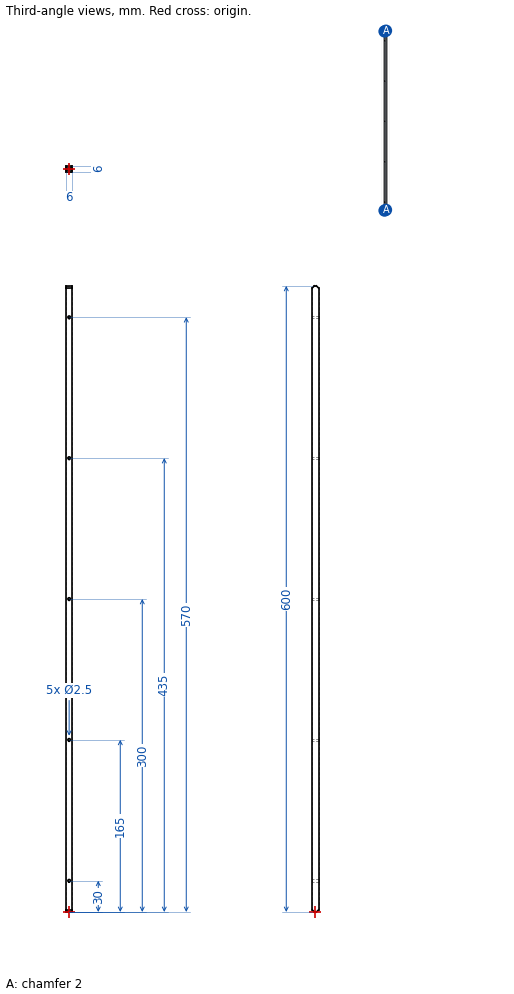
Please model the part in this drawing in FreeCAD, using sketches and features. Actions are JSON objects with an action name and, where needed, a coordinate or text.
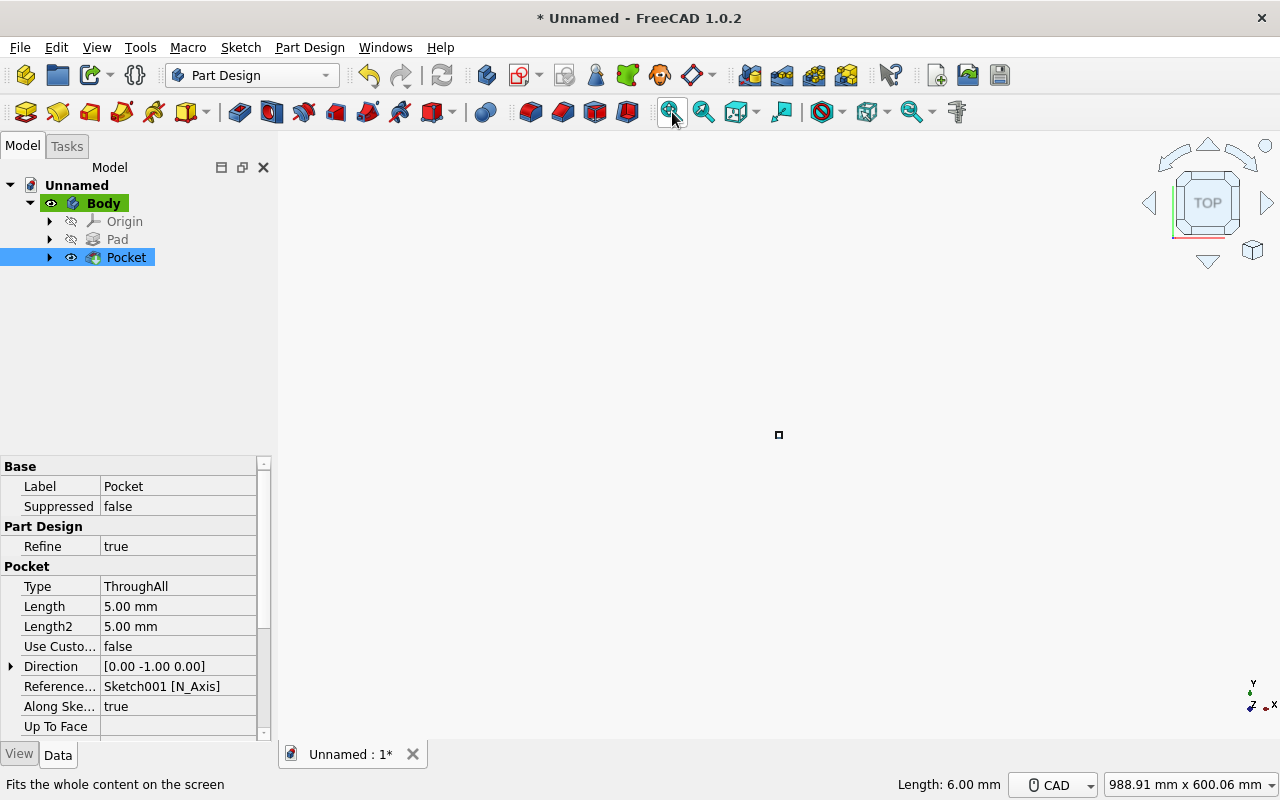
{"action": "left_click", "coordinate": [672, 112]}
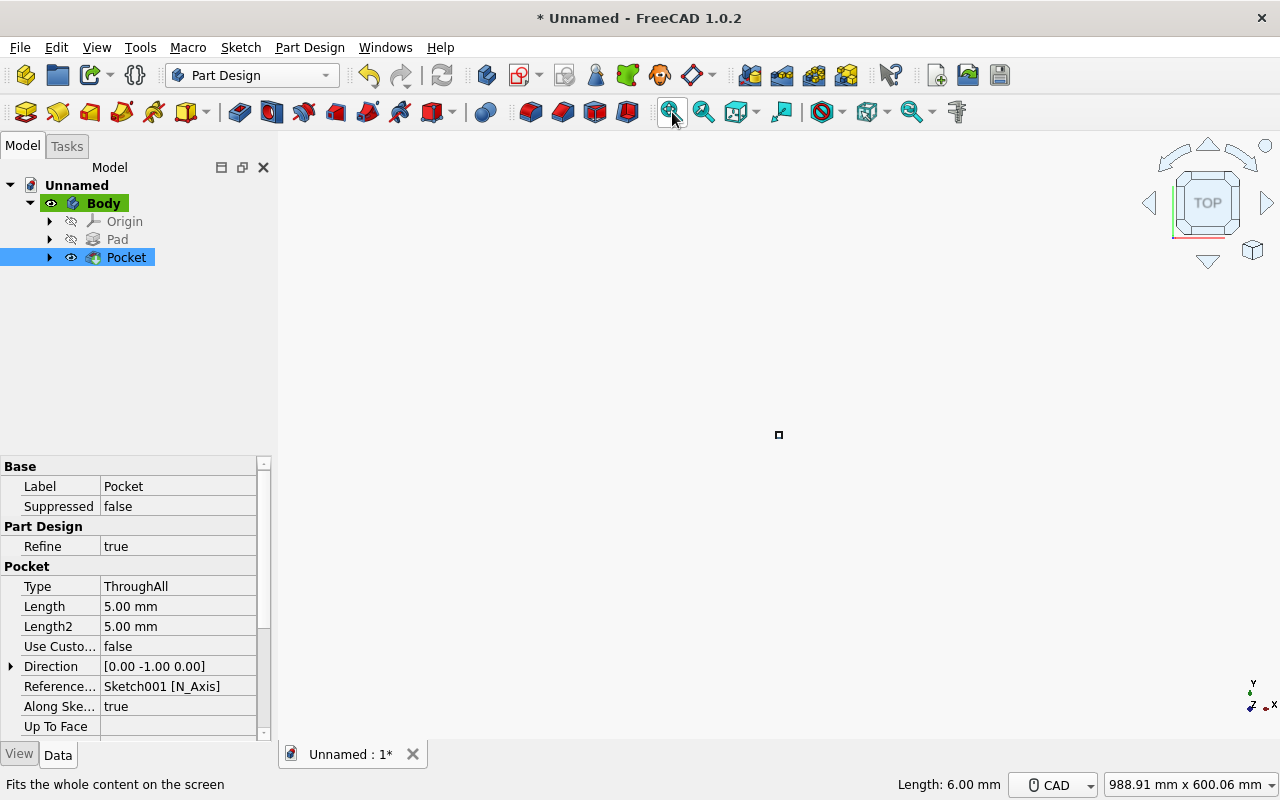
{"action": "scroll", "coordinate": [779, 437], "scroll_direction": "up", "scroll_amount": 10}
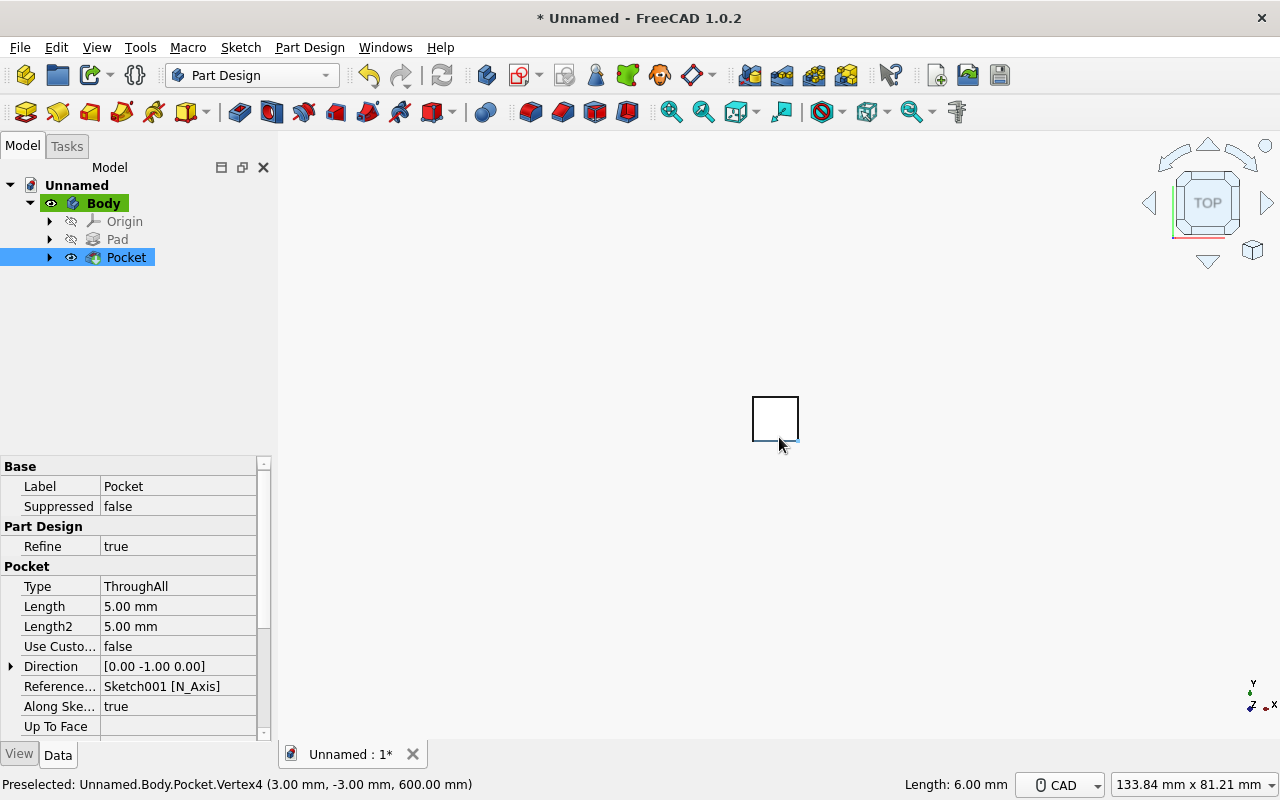
{"action": "left_click", "coordinate": [776, 396], "text": "ctrl"}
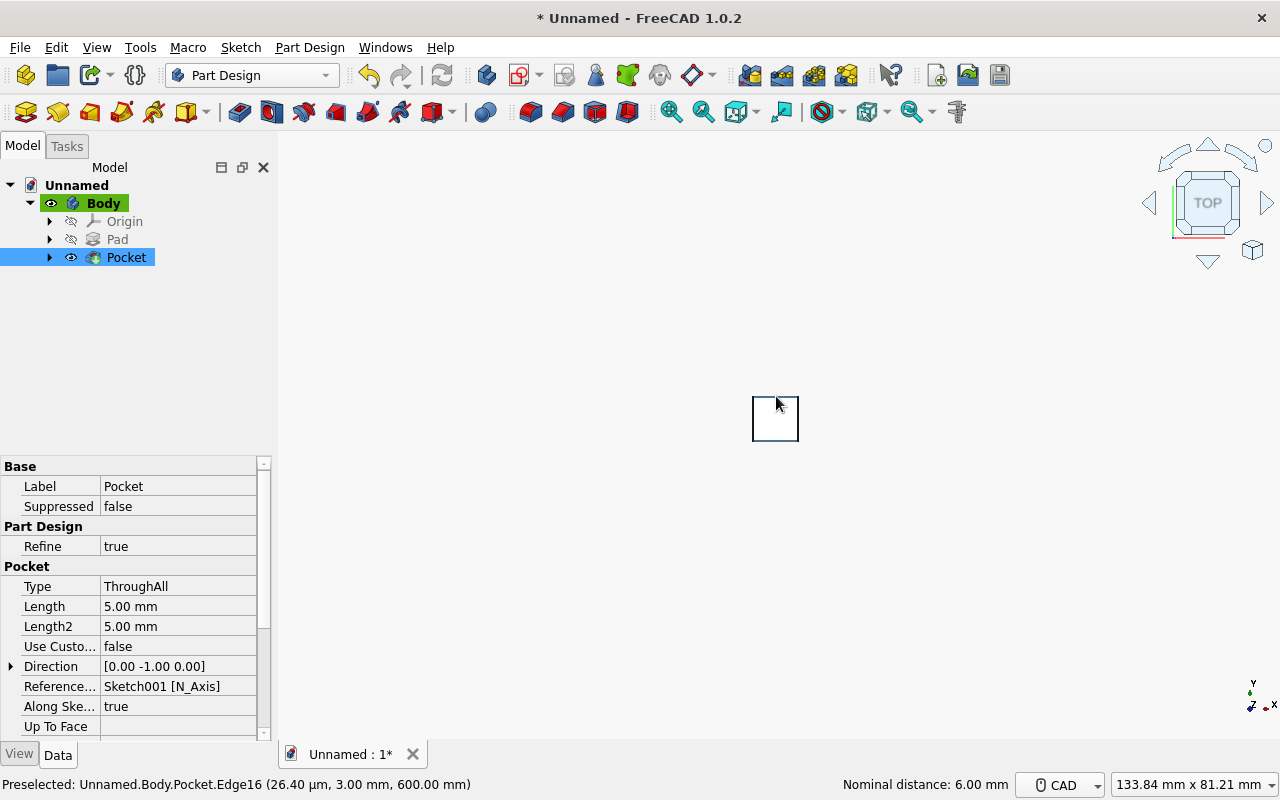
{"action": "left_click", "coordinate": [672, 112]}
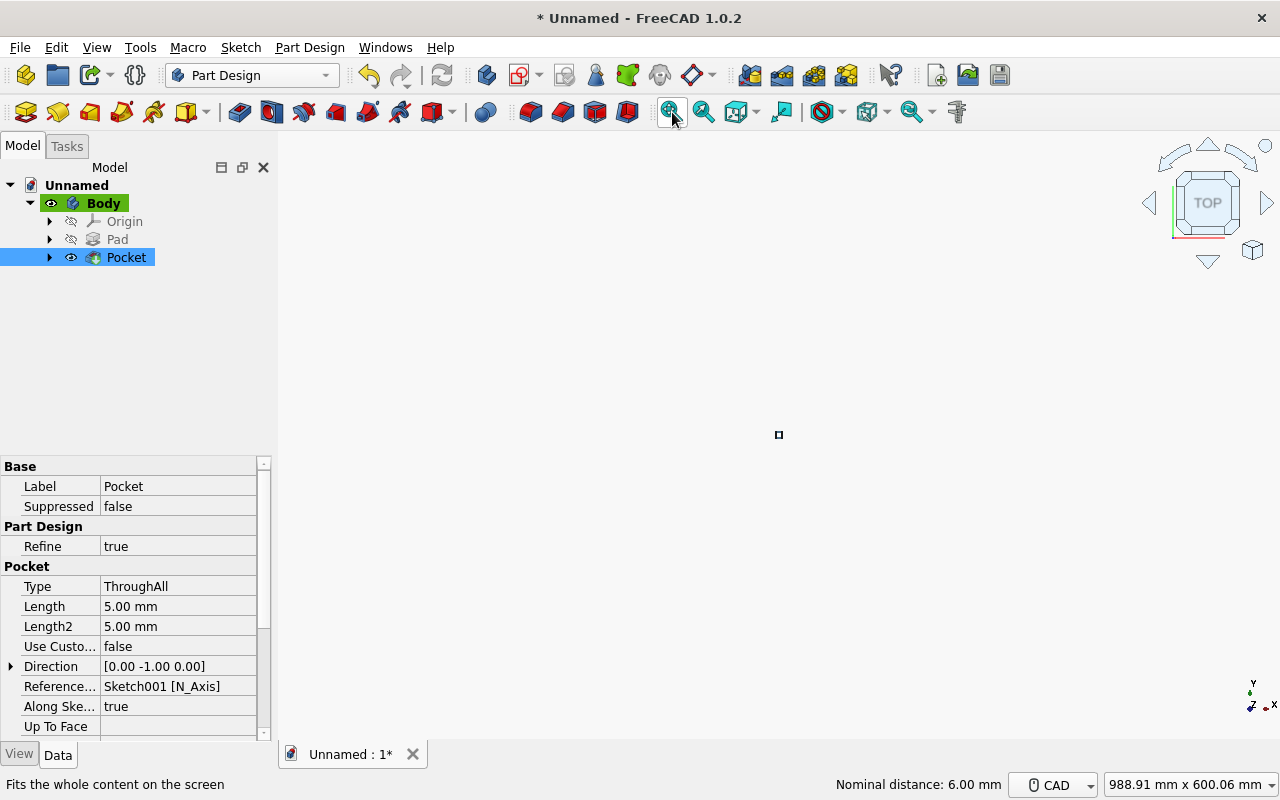
{"action": "key", "text": "1"}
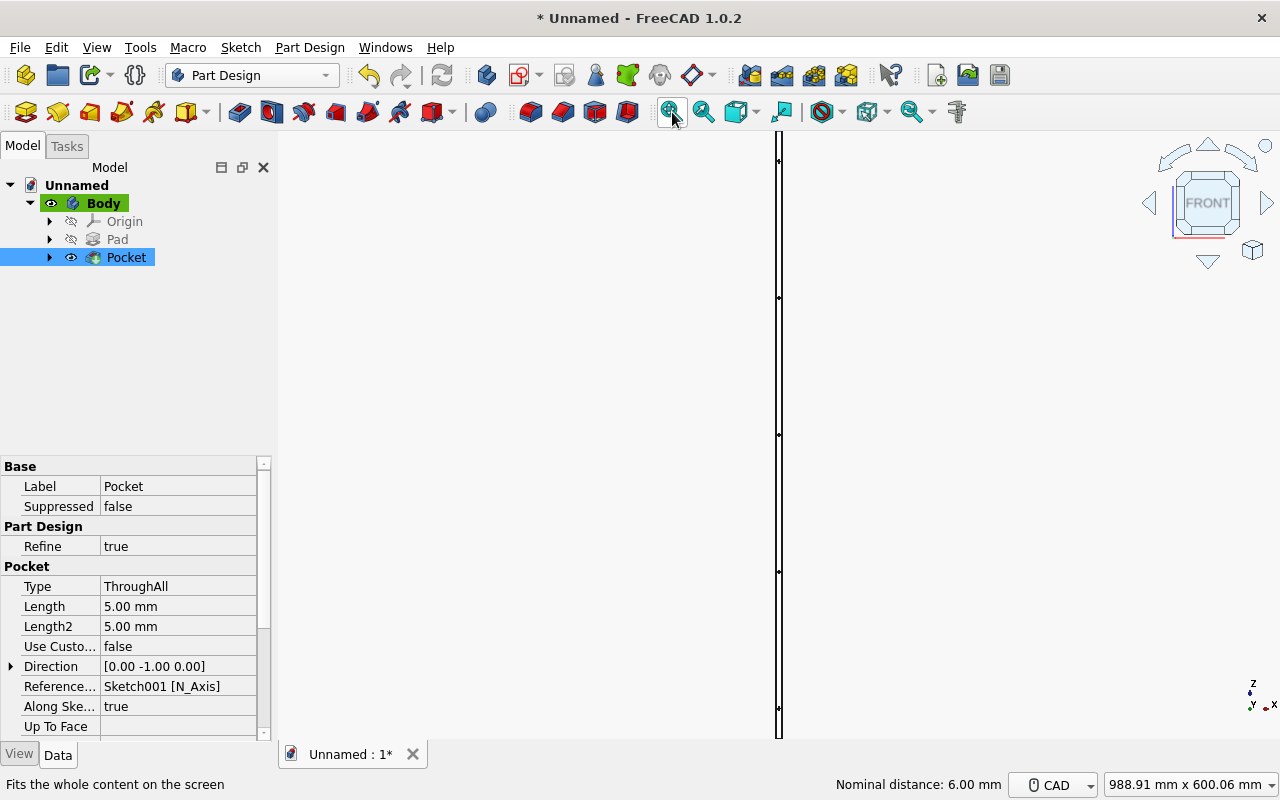
{"action": "left_click", "coordinate": [672, 112]}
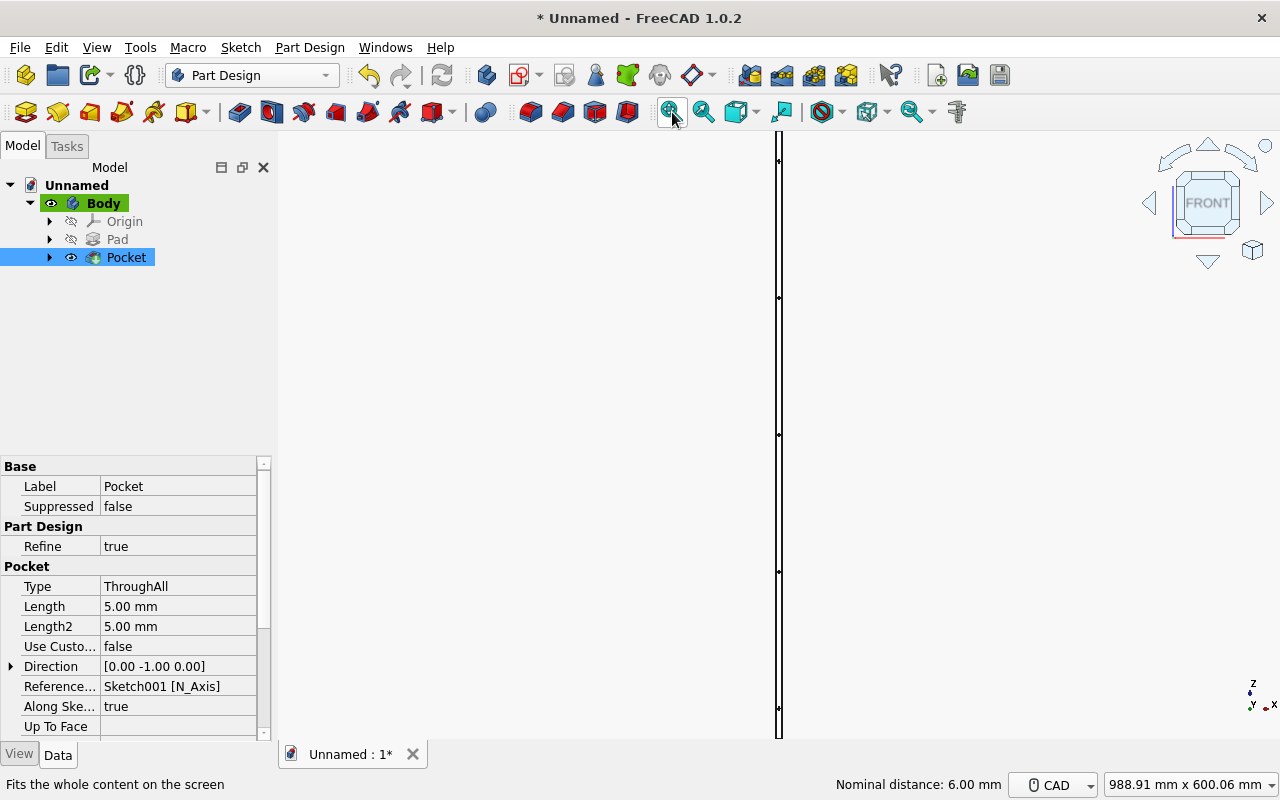
{"action": "key", "text": "3"}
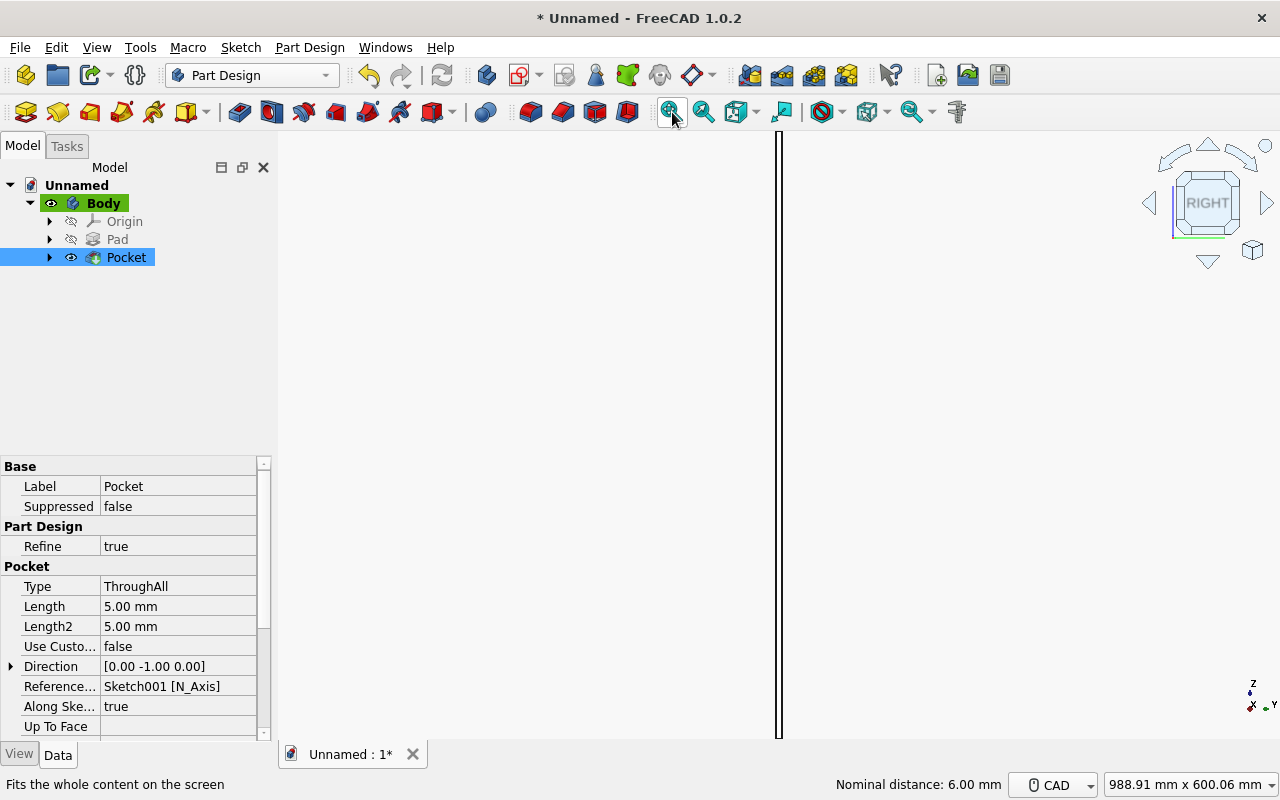
{"action": "left_click", "coordinate": [672, 112]}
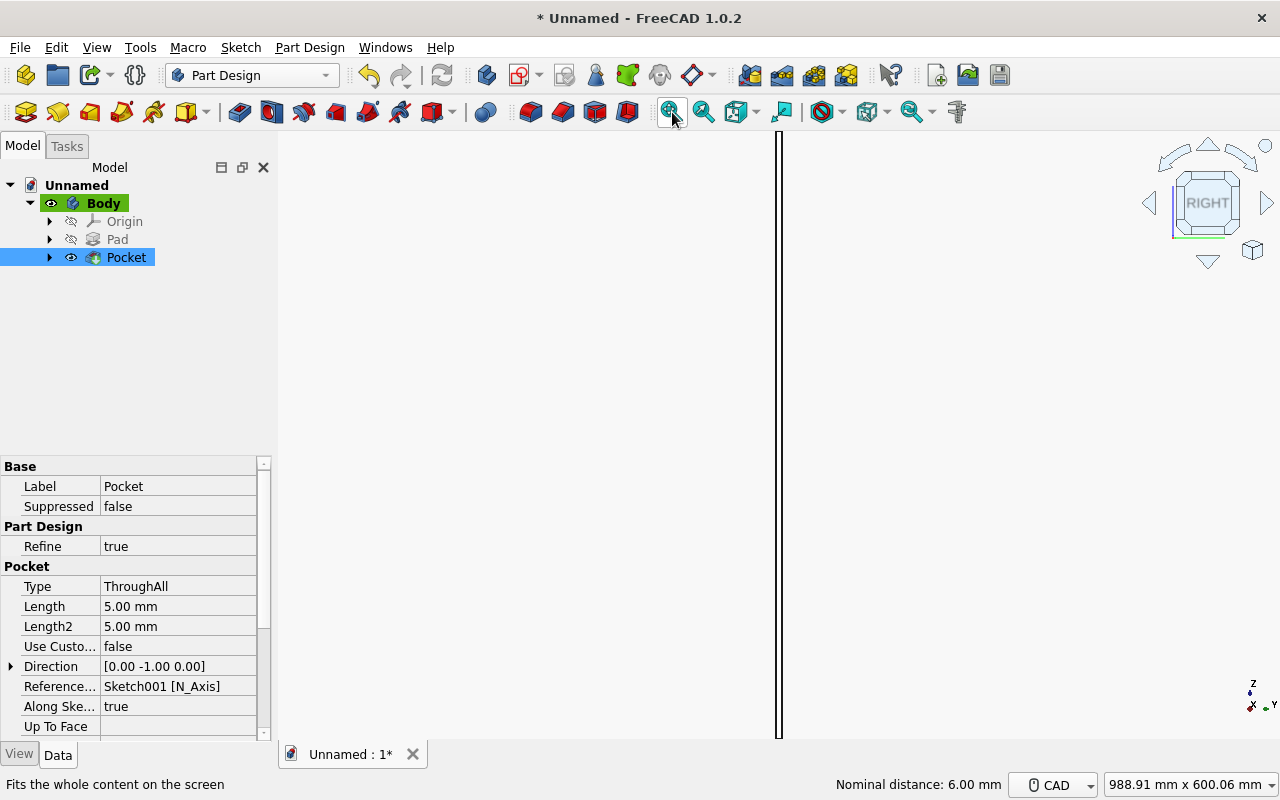
{"action": "key", "text": "5"}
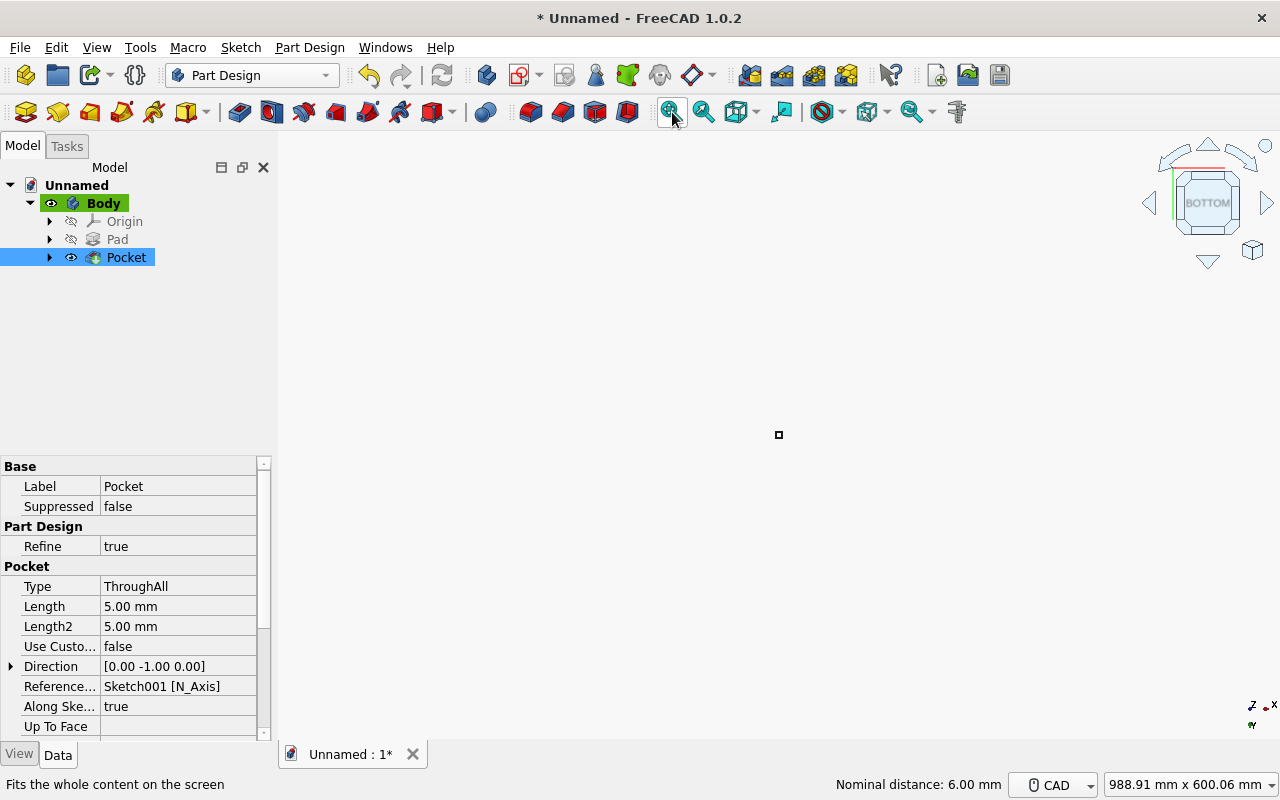
{"action": "left_click", "coordinate": [672, 112]}